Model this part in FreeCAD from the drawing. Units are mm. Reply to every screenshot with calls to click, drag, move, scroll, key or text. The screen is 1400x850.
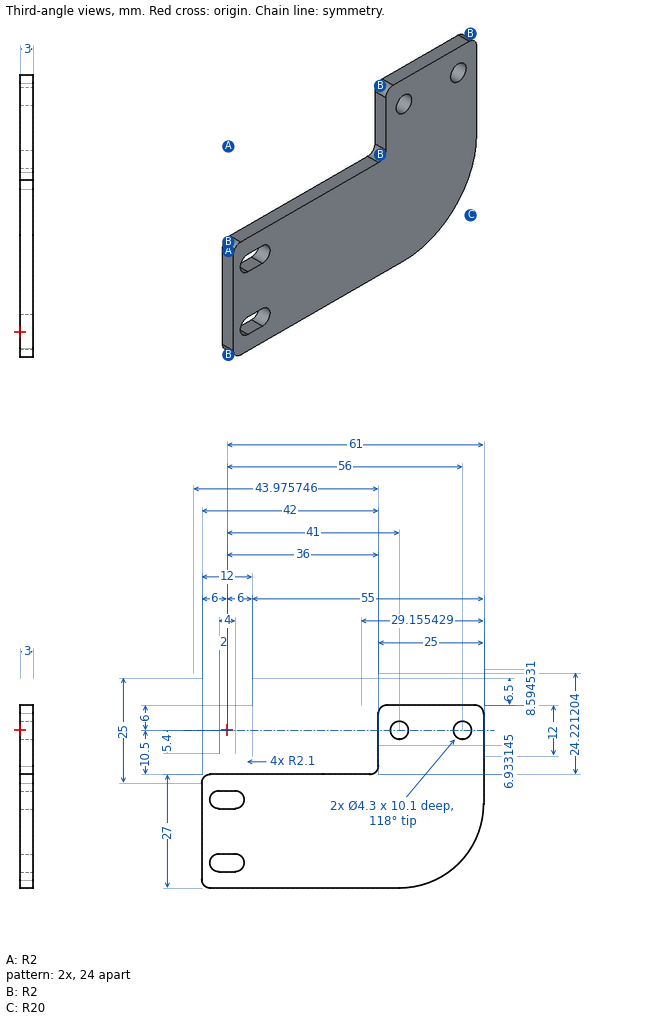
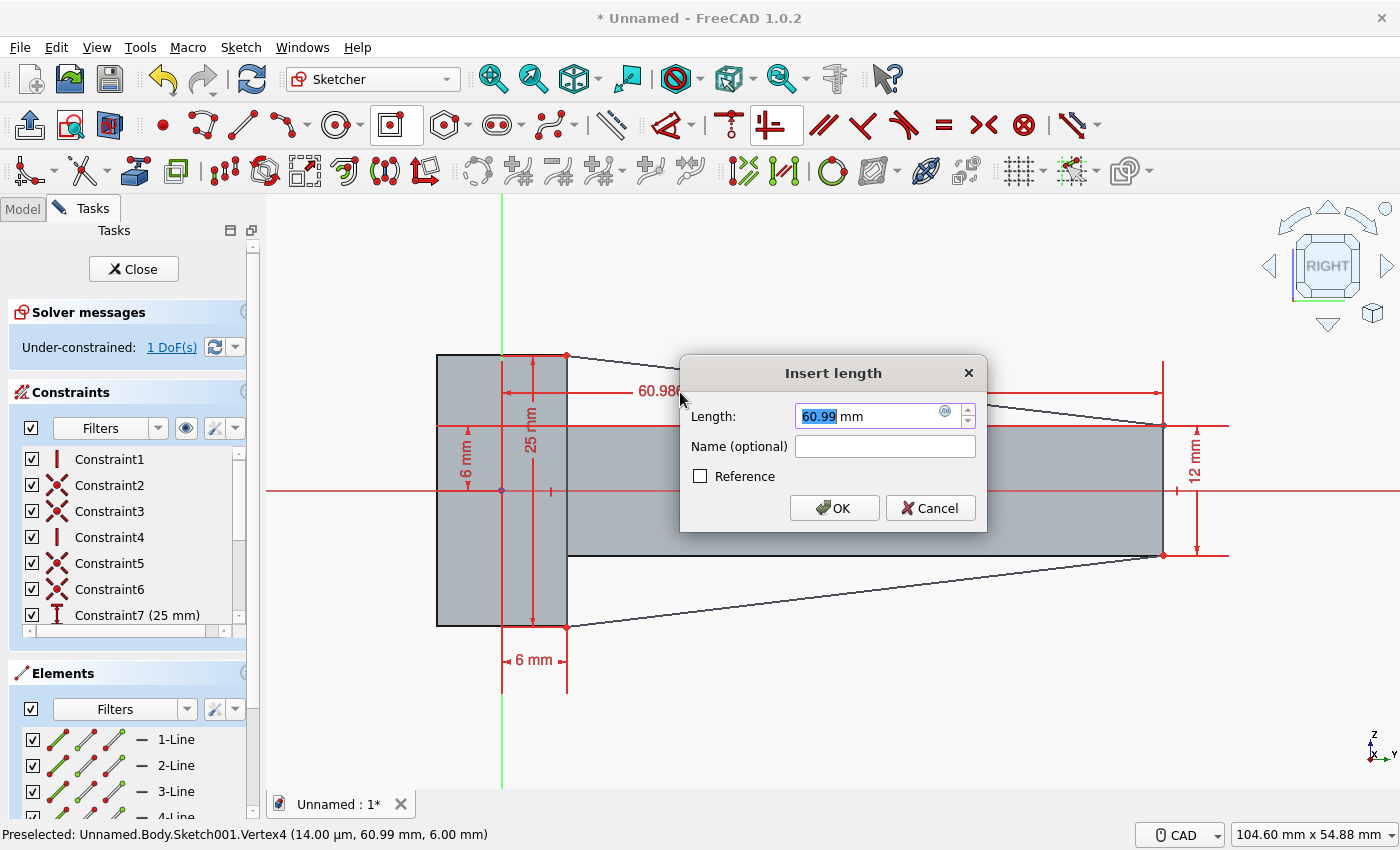
text(61)
key(Return)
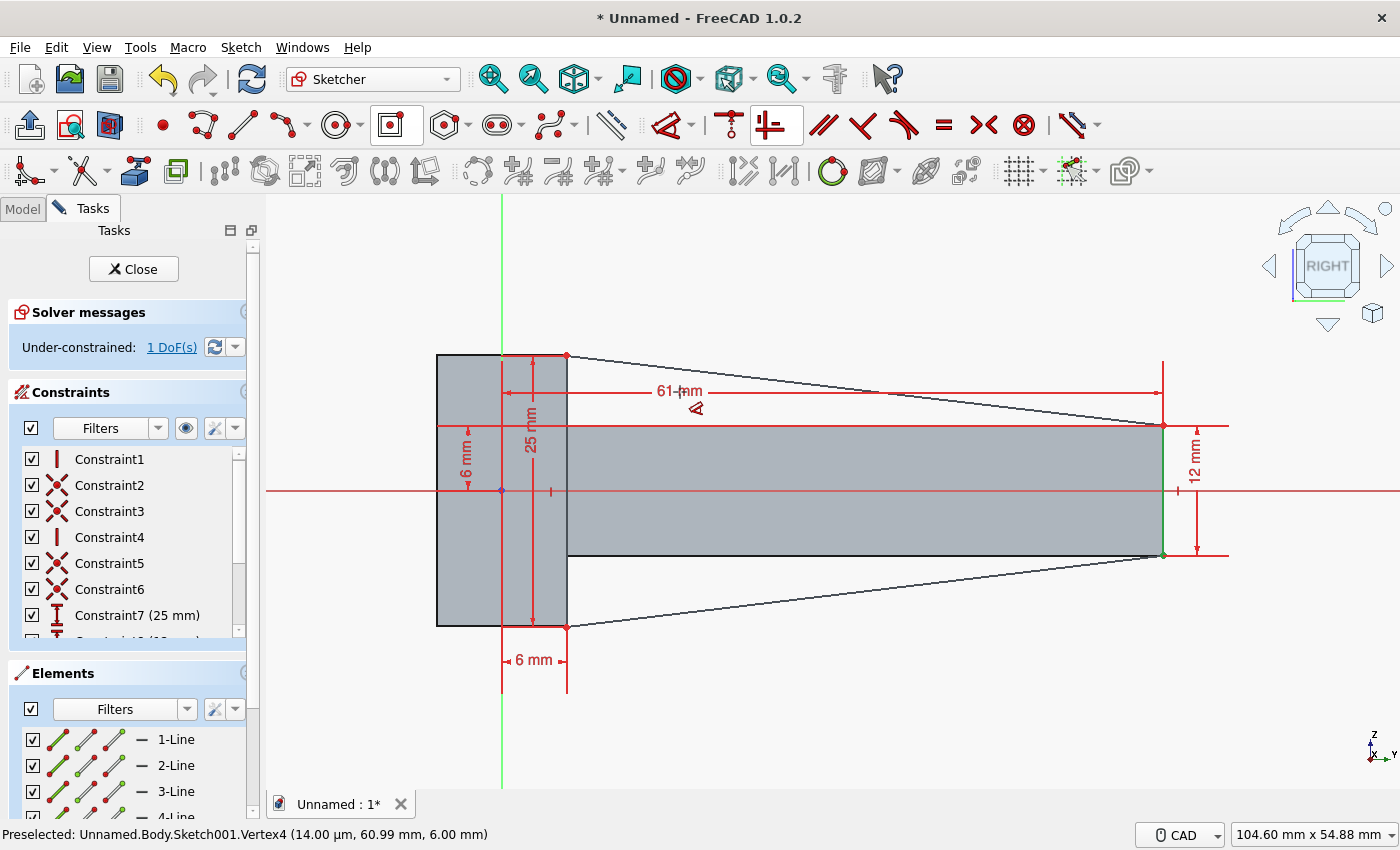
click(746, 377)
click(1197, 391)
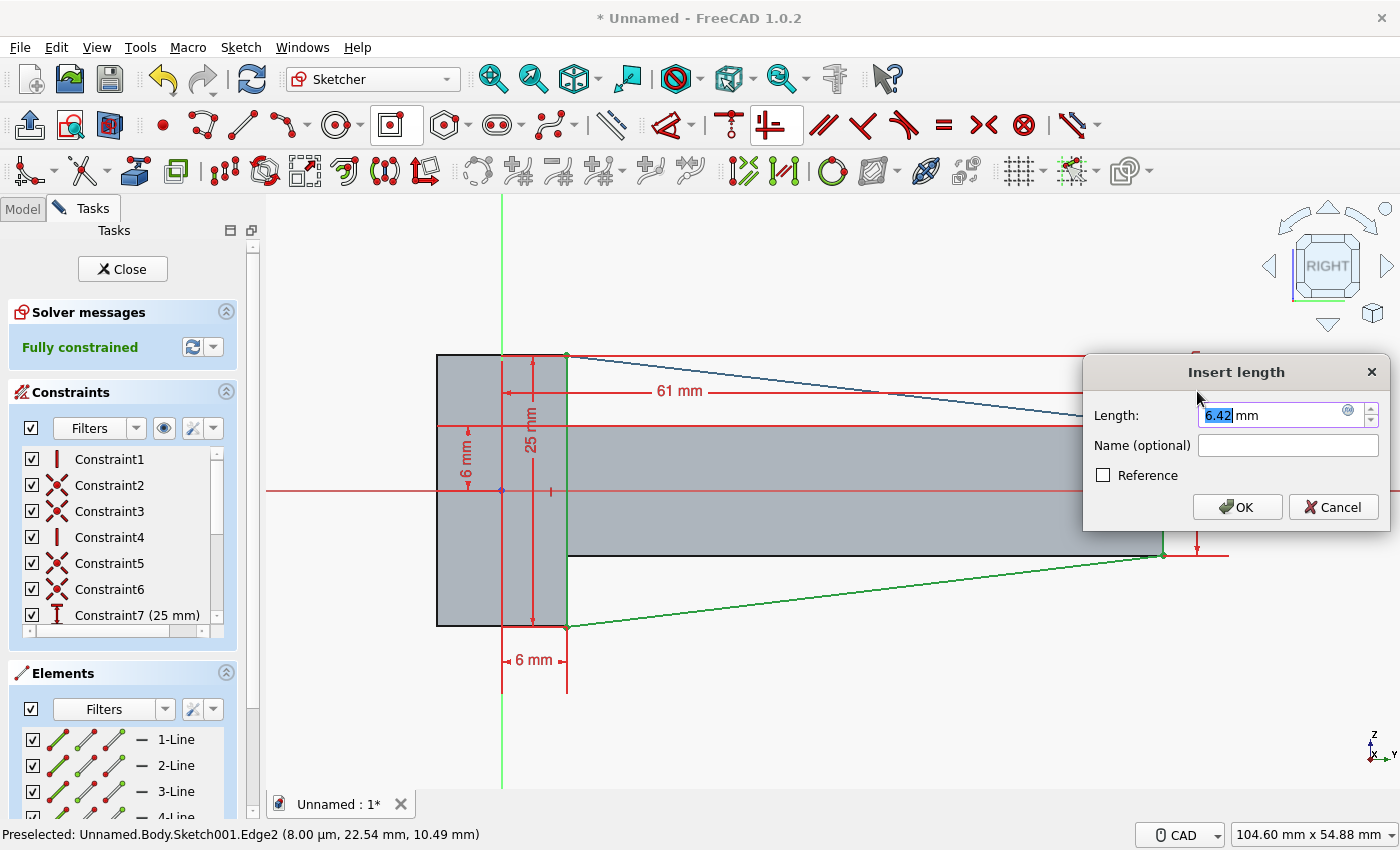
text(6.5)
key(Return)
key(Escape)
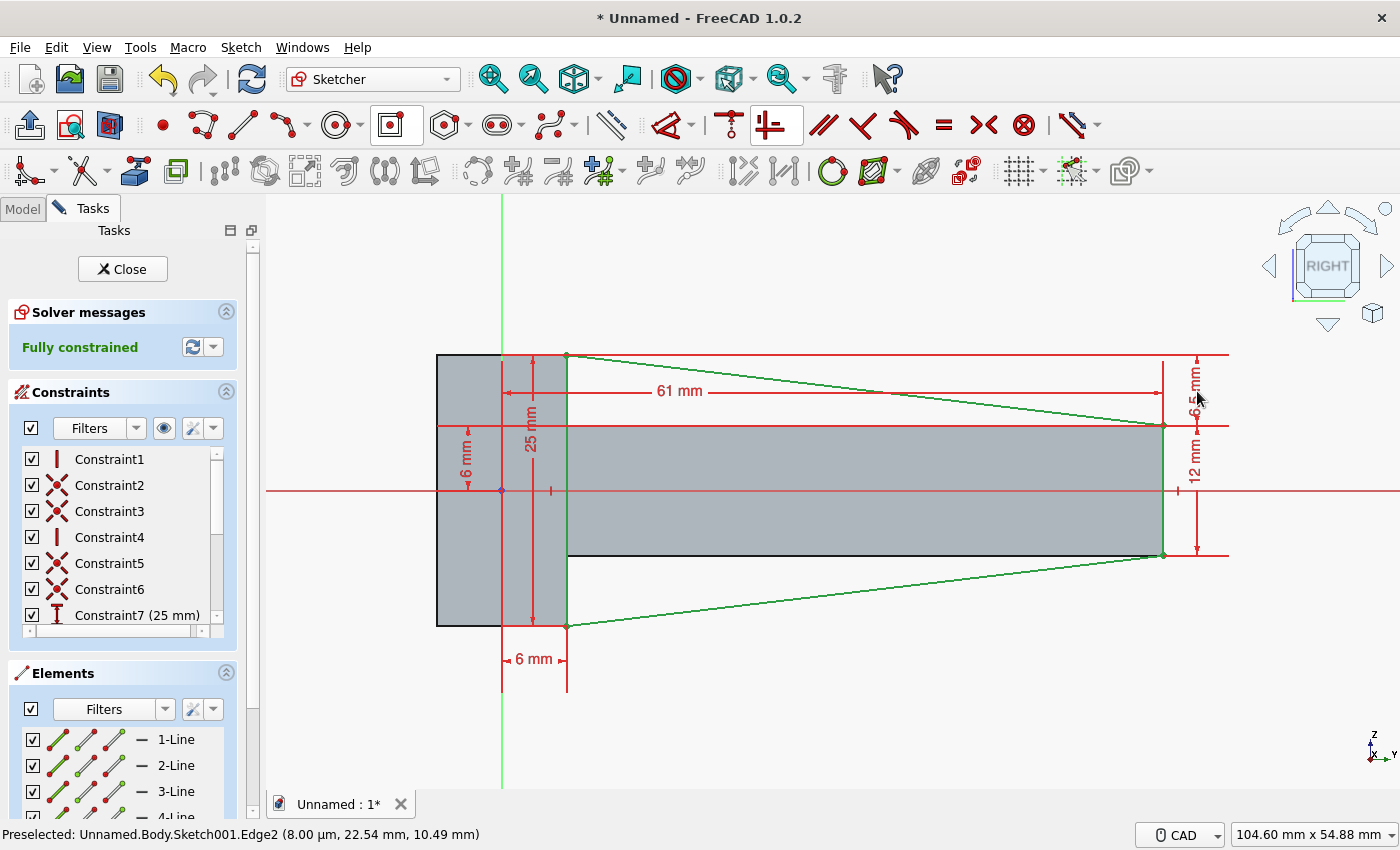
click(123, 269)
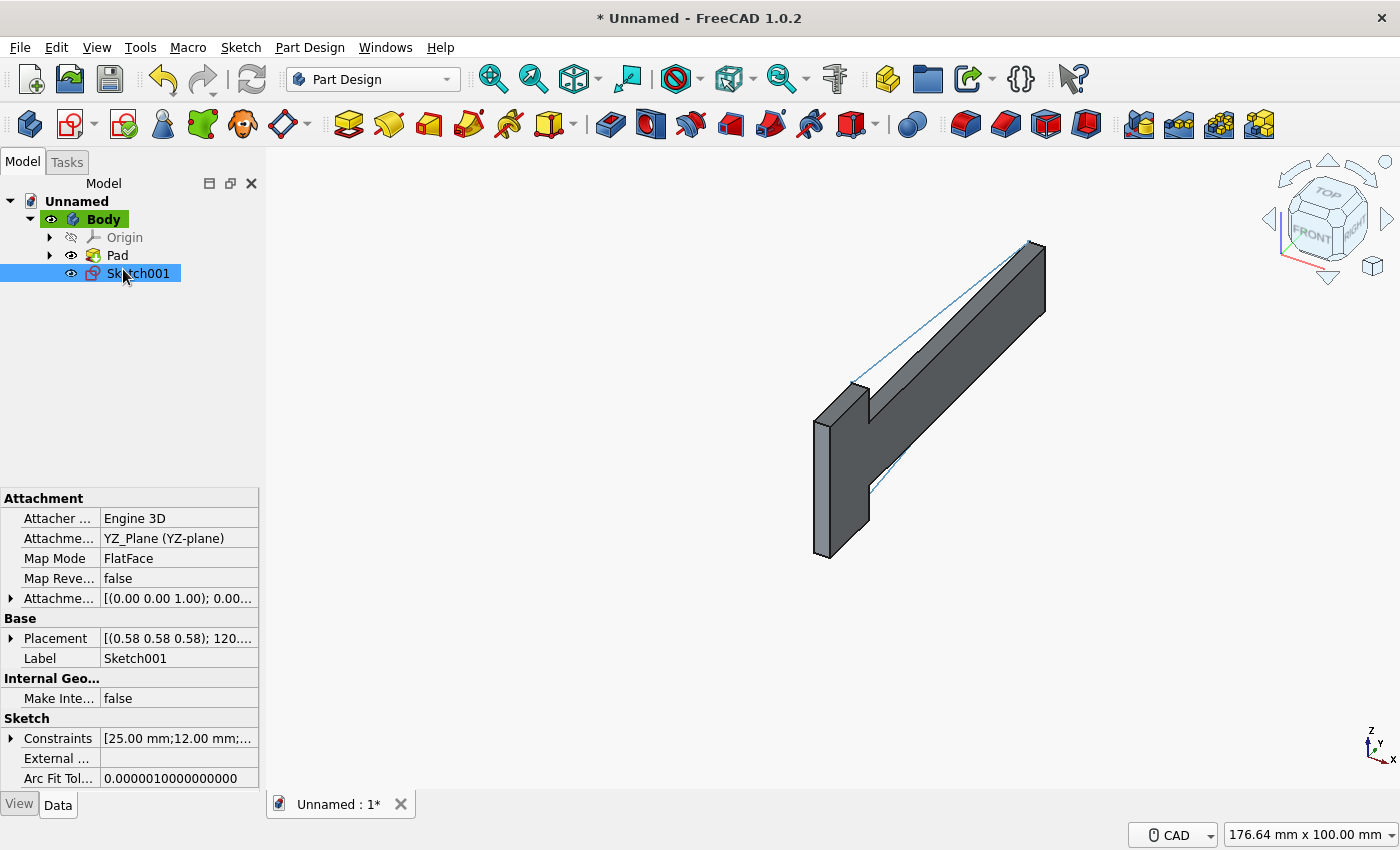
click(350, 124)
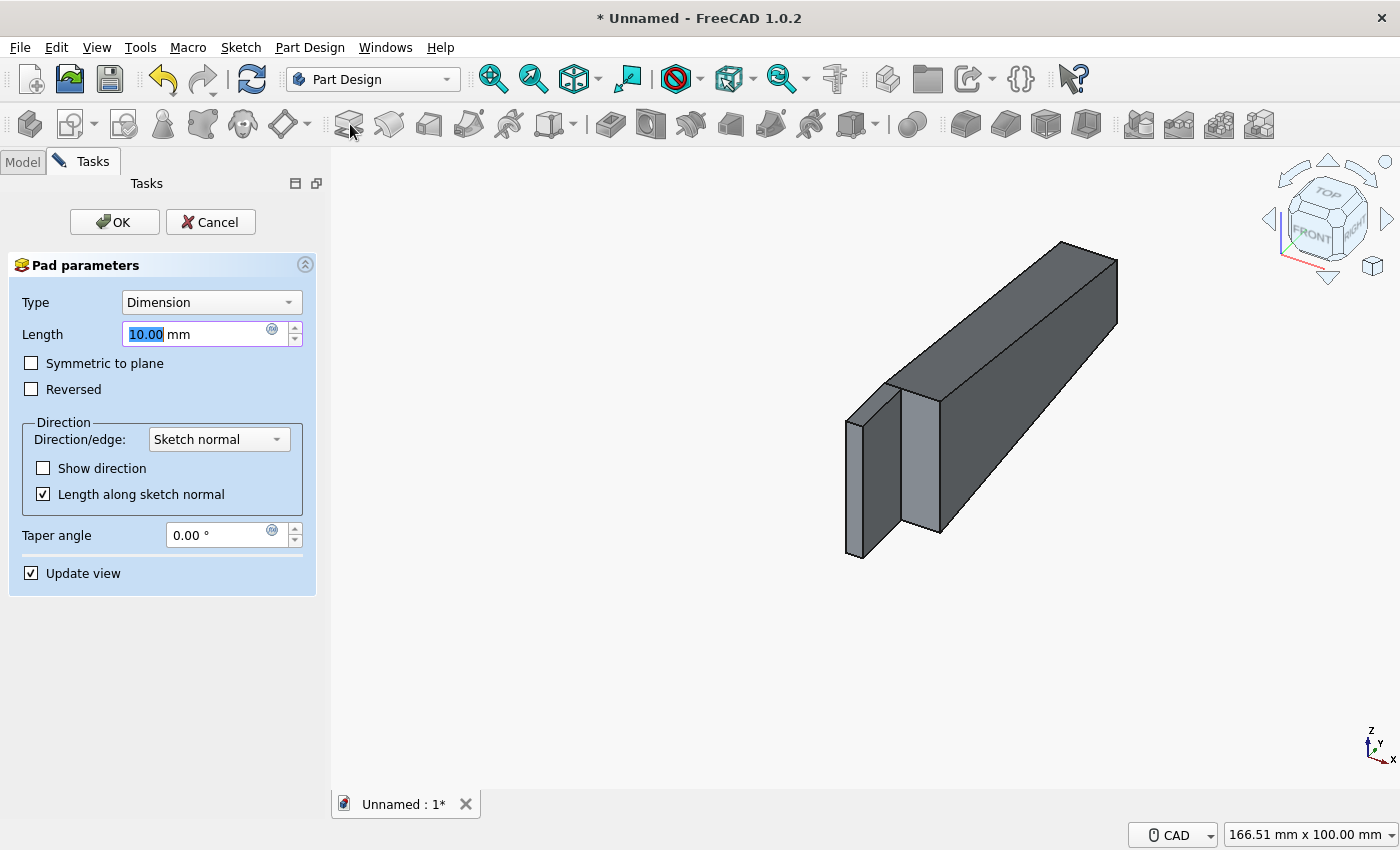
text(3)
key(Tab)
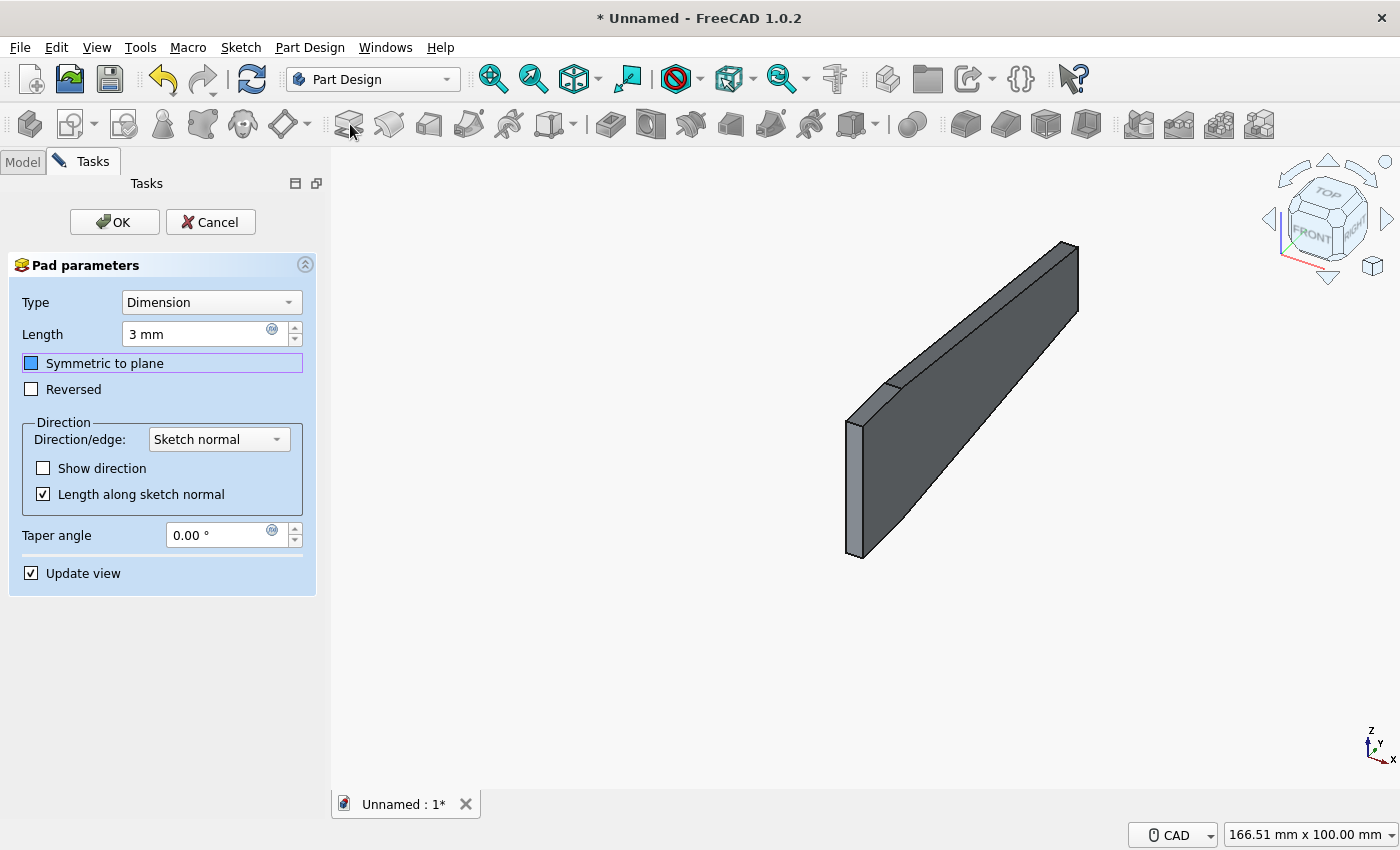
click(115, 222)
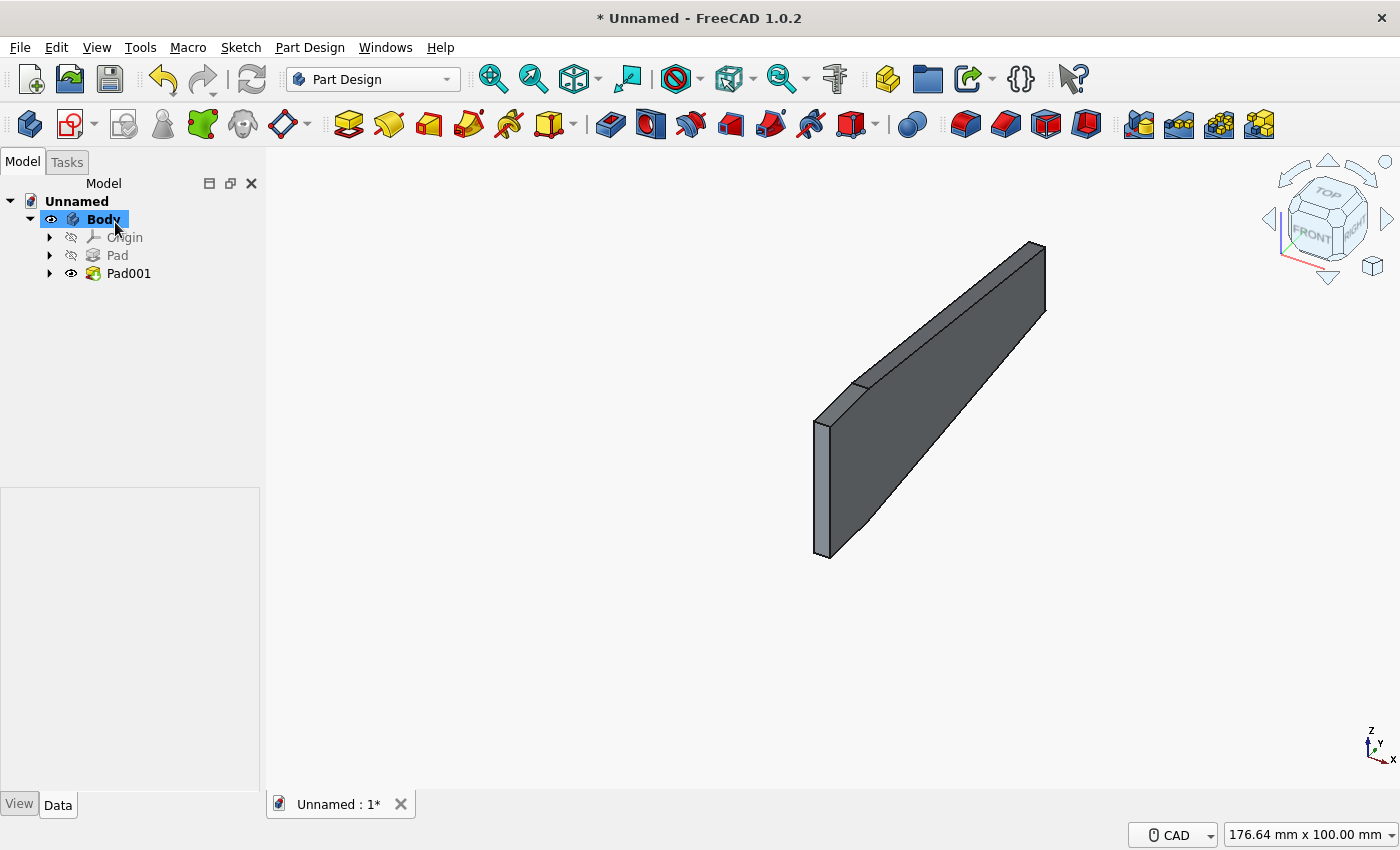
click(70, 124)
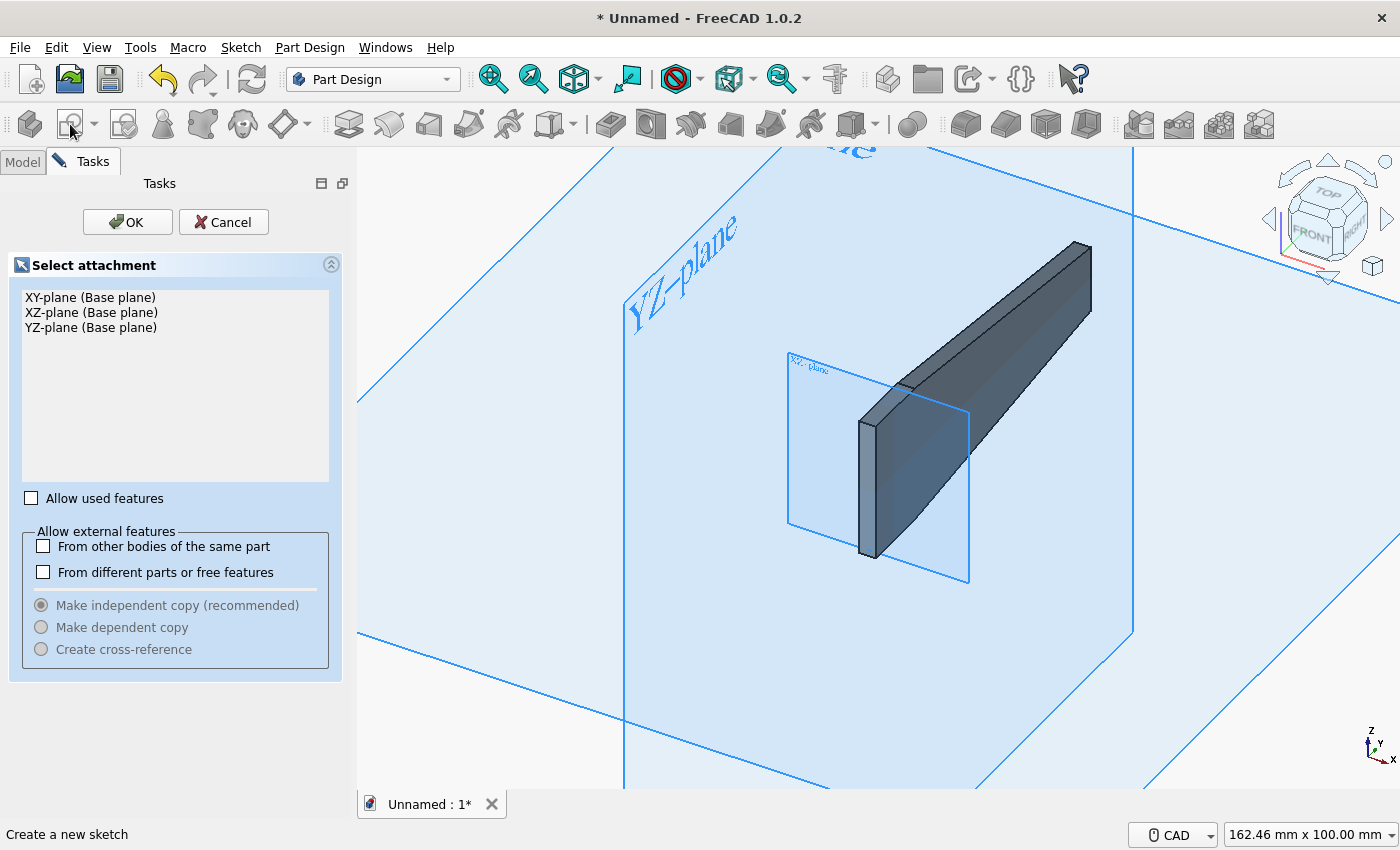
click(82, 328)